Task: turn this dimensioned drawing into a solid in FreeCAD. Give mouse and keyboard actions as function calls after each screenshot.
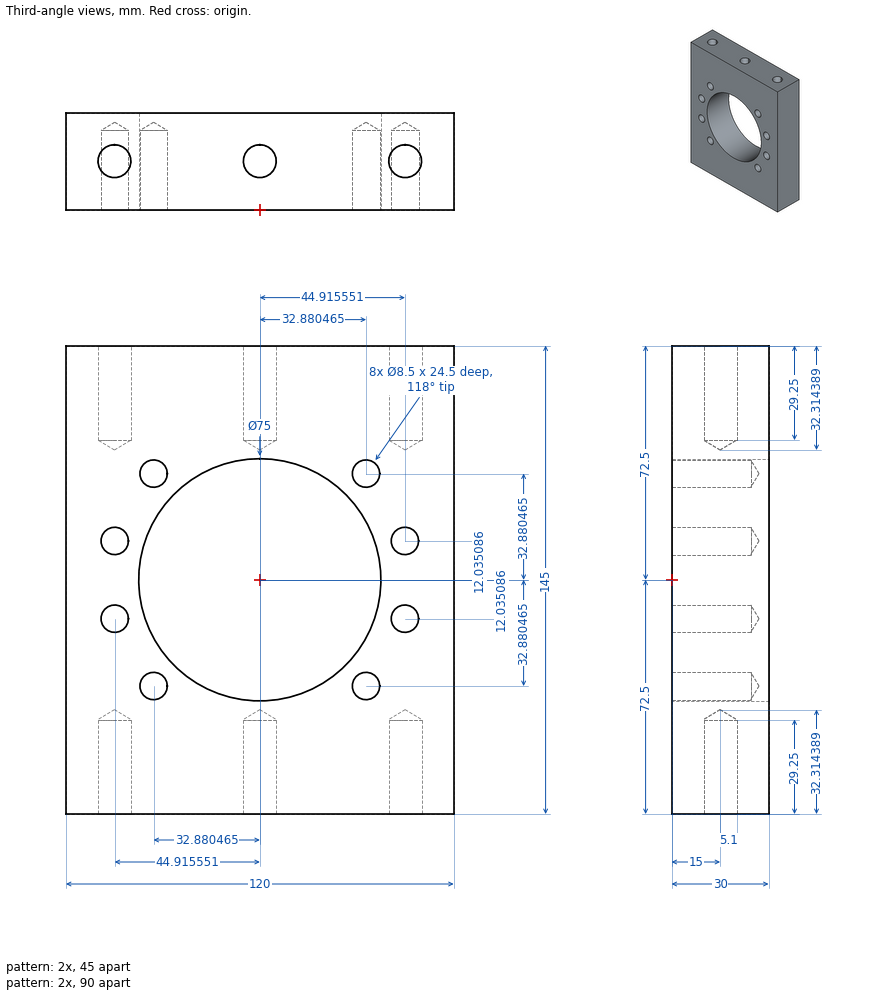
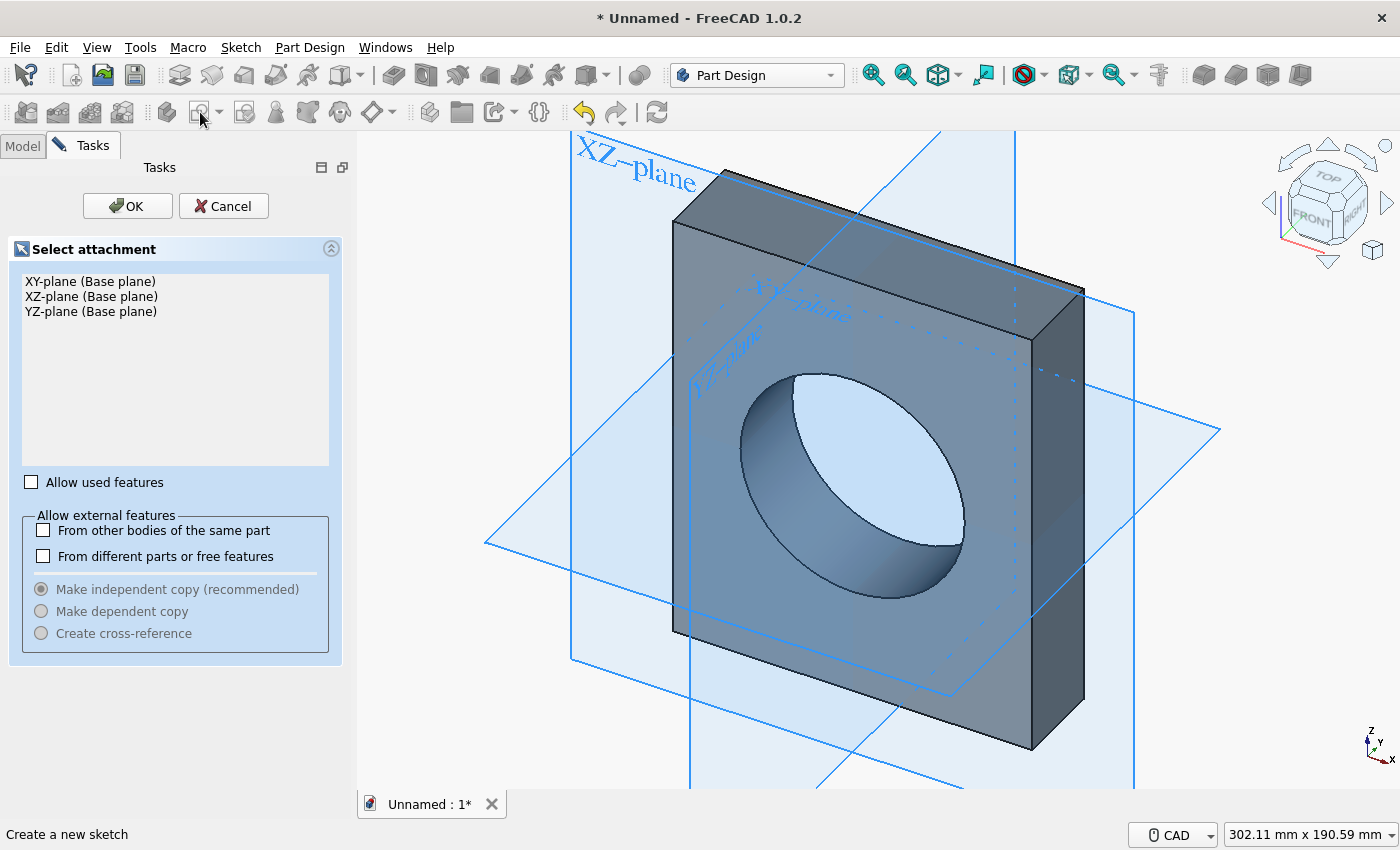
click(82, 296)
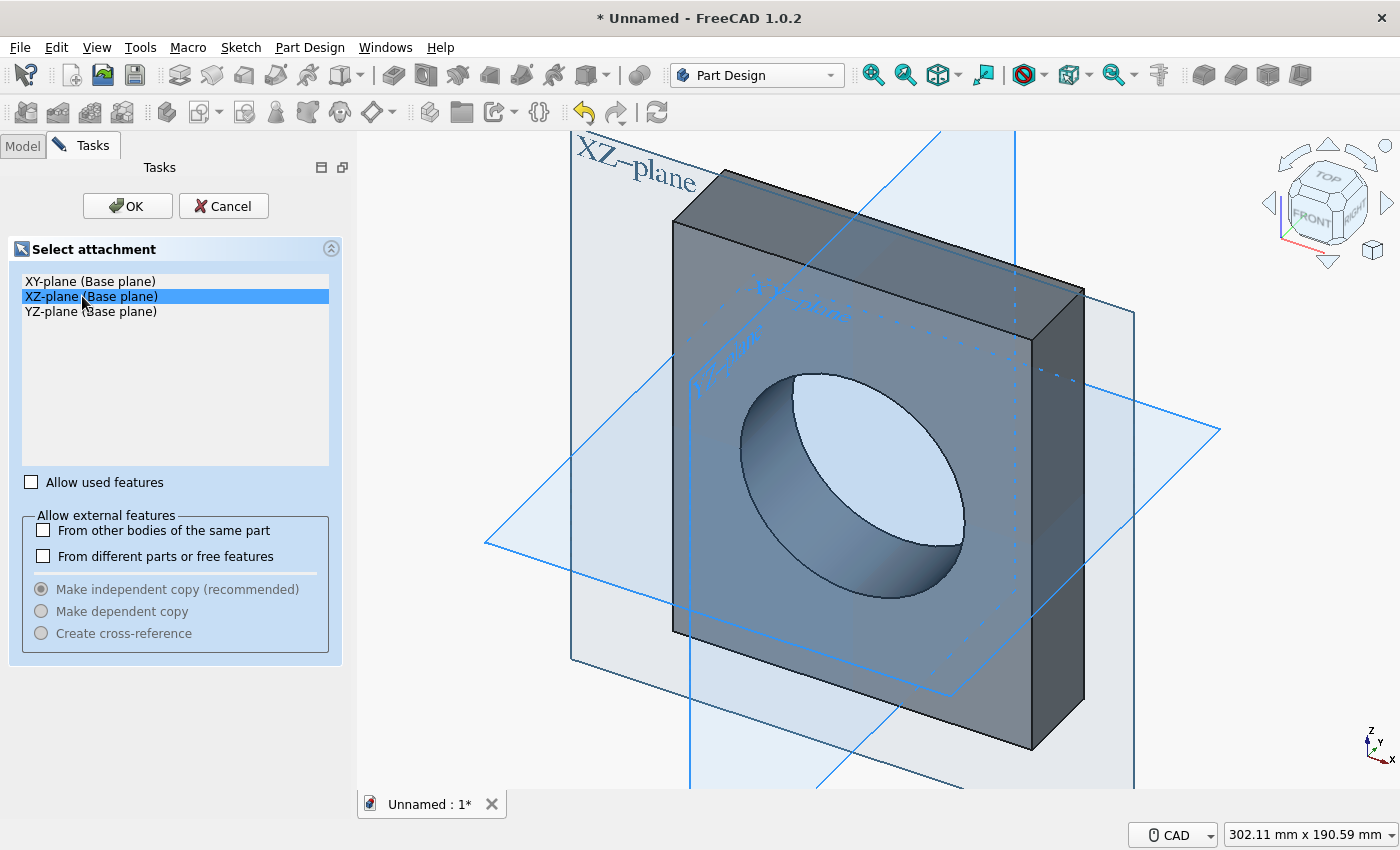
click(128, 206)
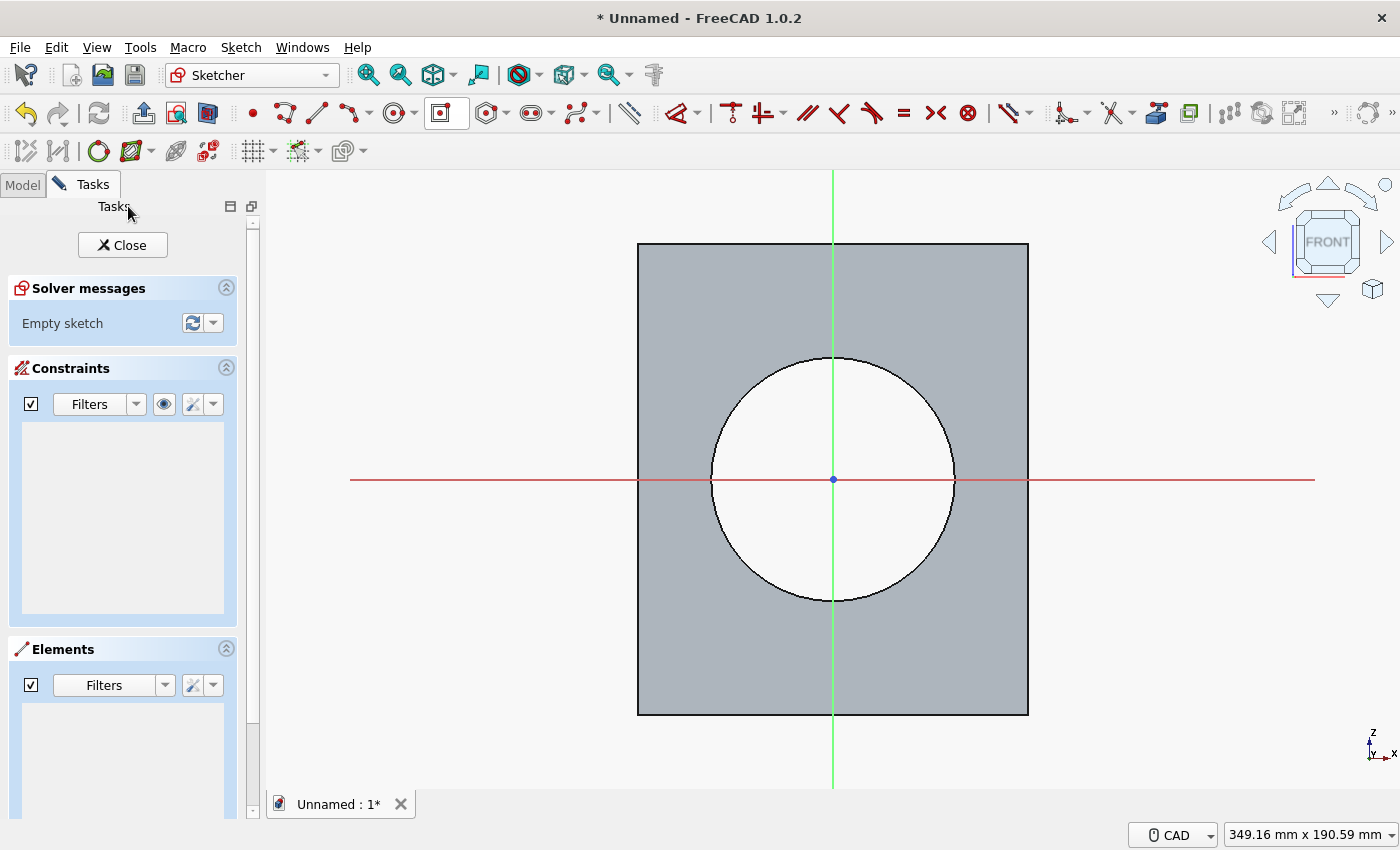
scroll(972, 480, up, 2)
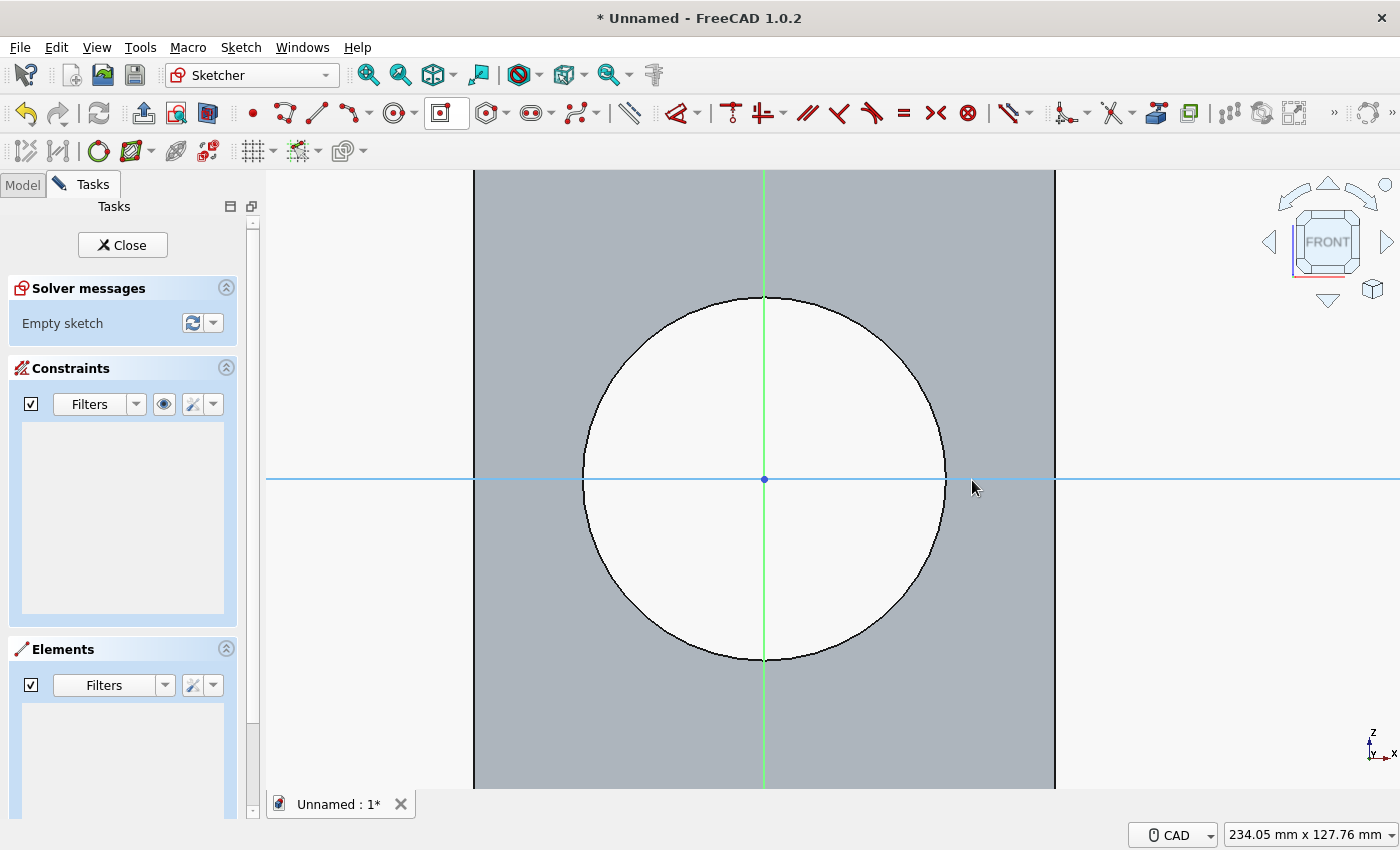
click(394, 114)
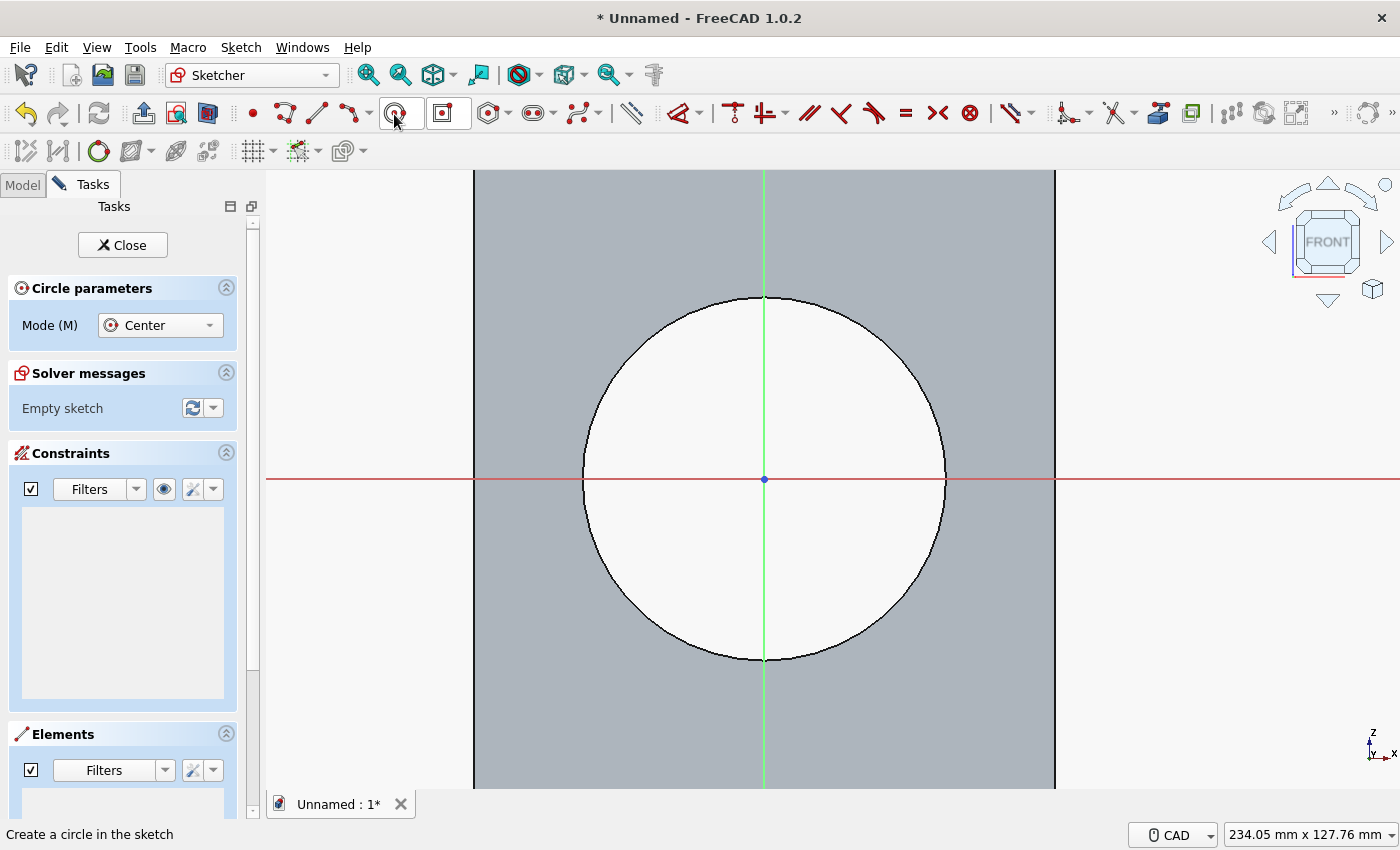
click(924, 320)
click(938, 305)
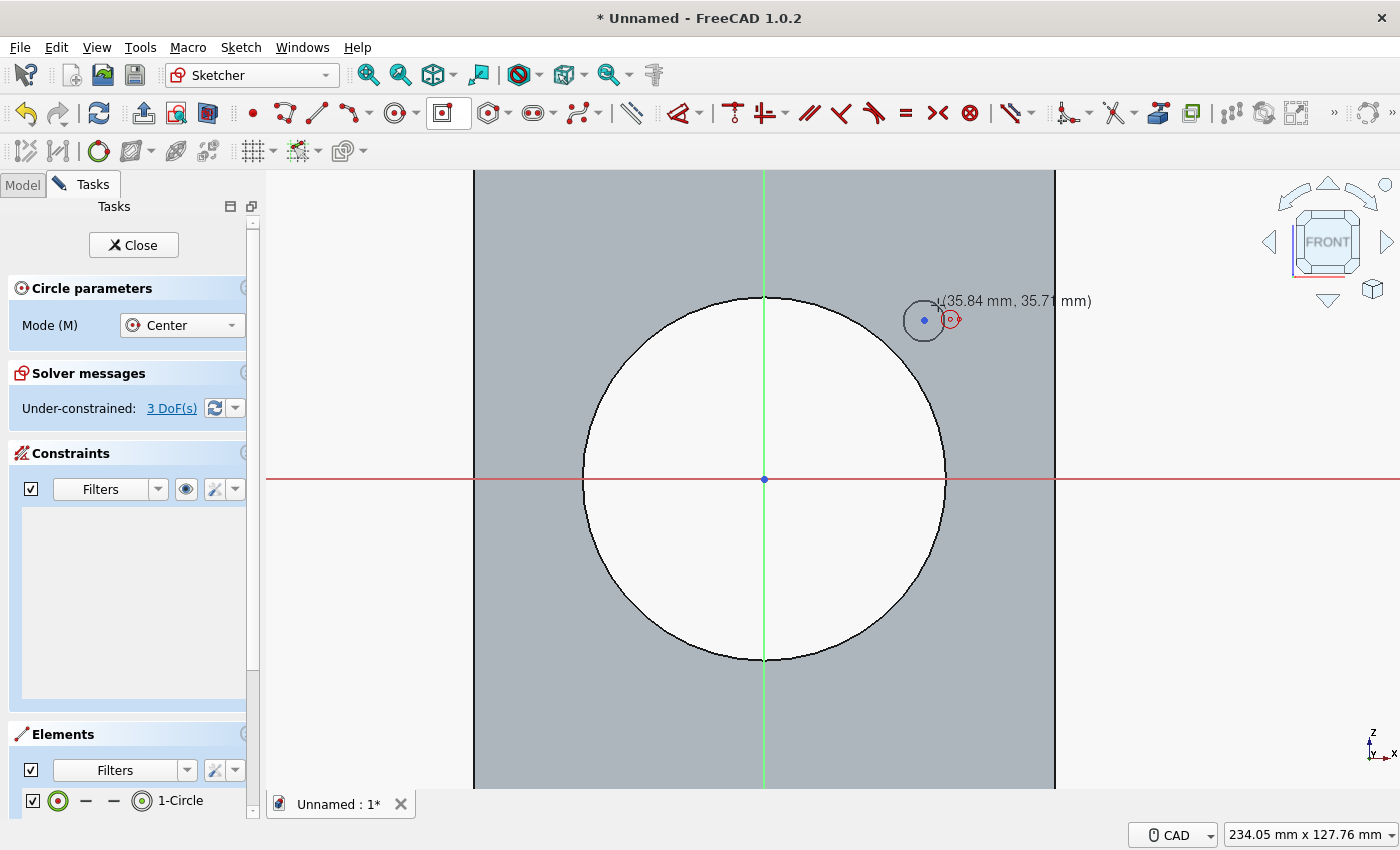
click(982, 421)
click(997, 406)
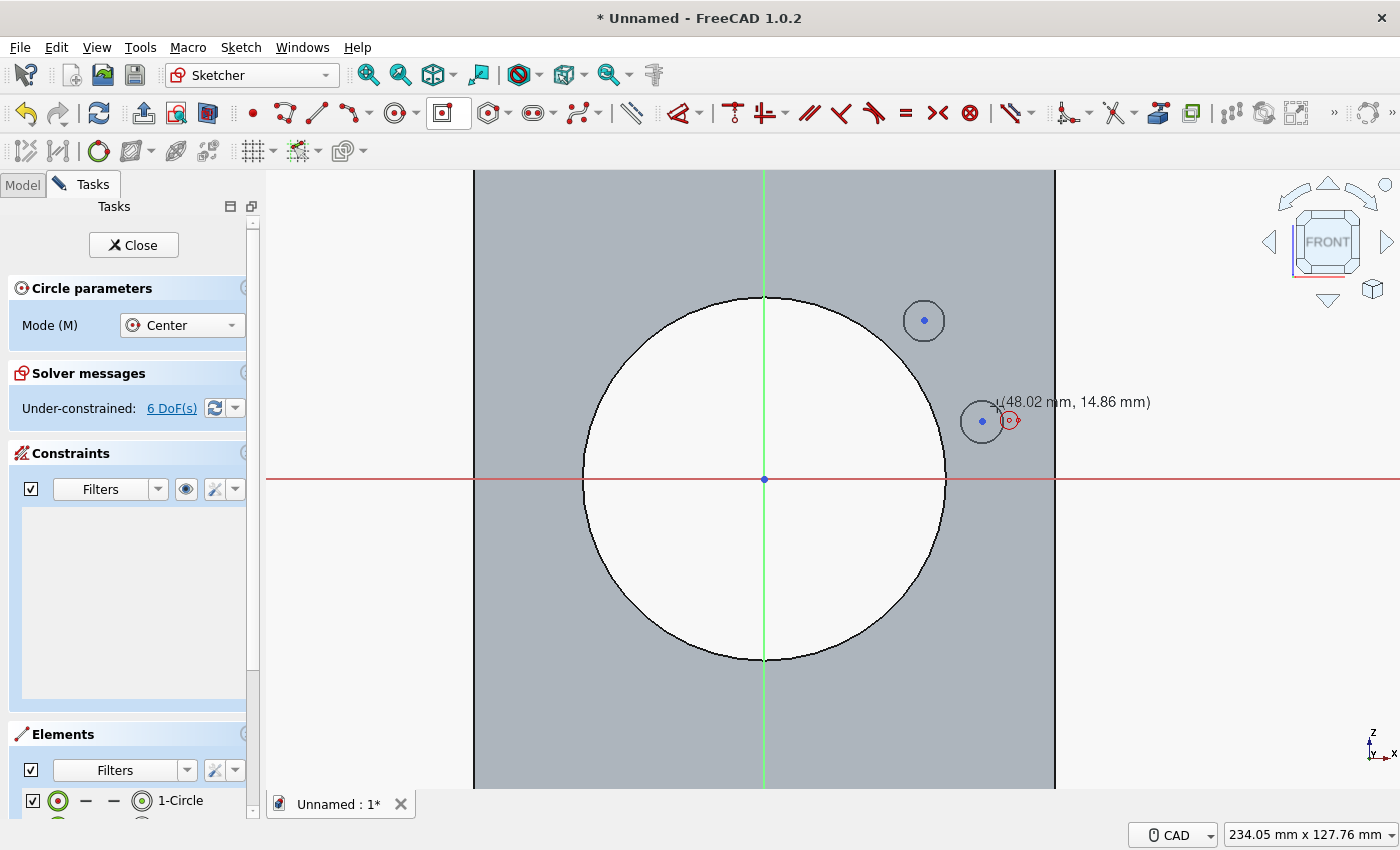
click(982, 537)
click(997, 523)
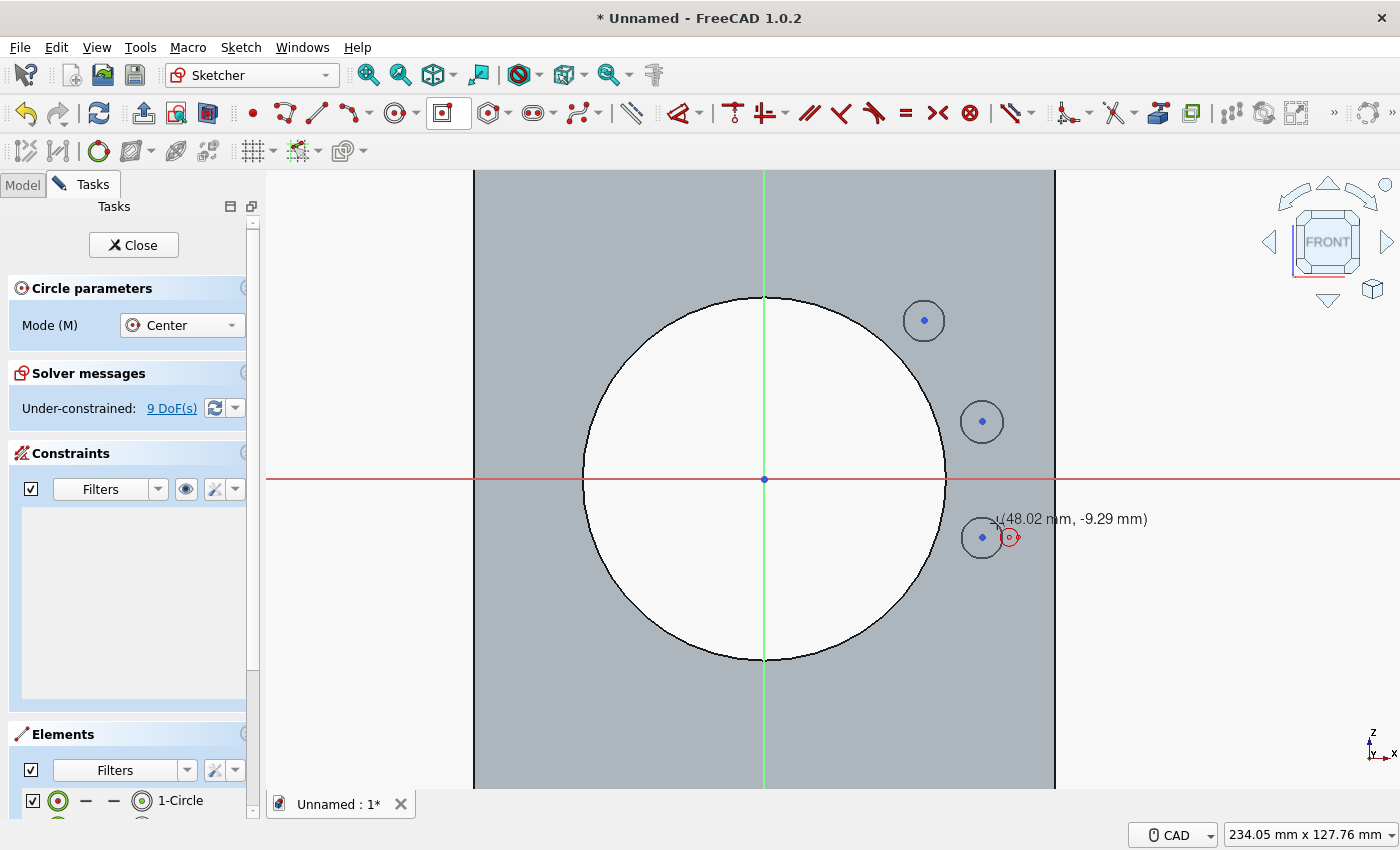
click(924, 638)
click(938, 624)